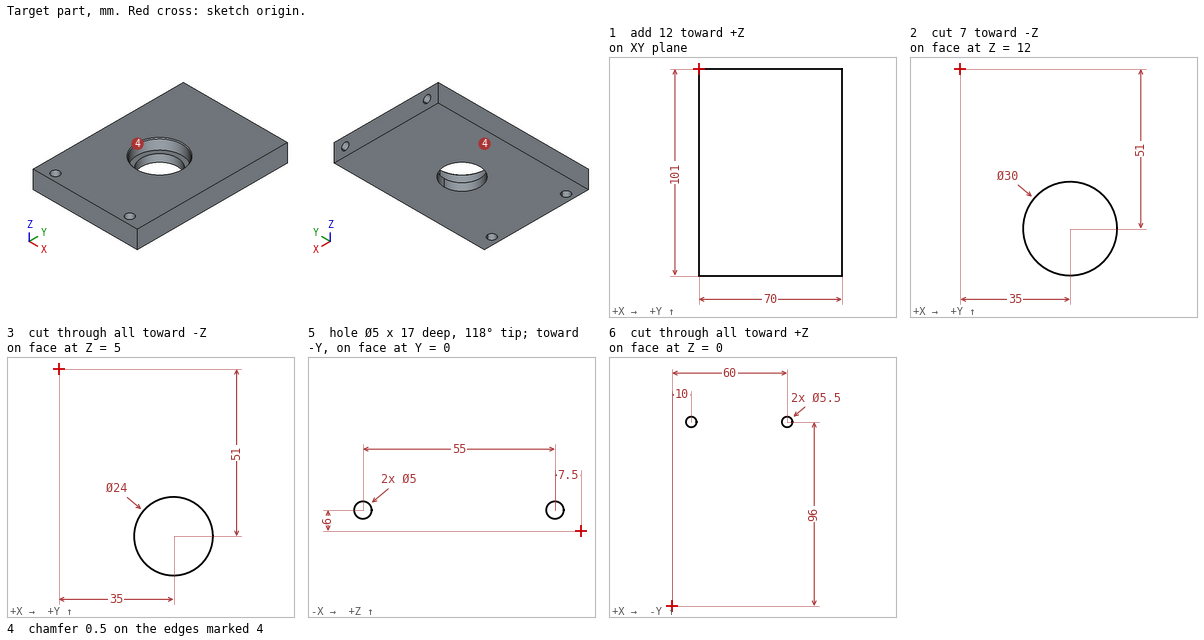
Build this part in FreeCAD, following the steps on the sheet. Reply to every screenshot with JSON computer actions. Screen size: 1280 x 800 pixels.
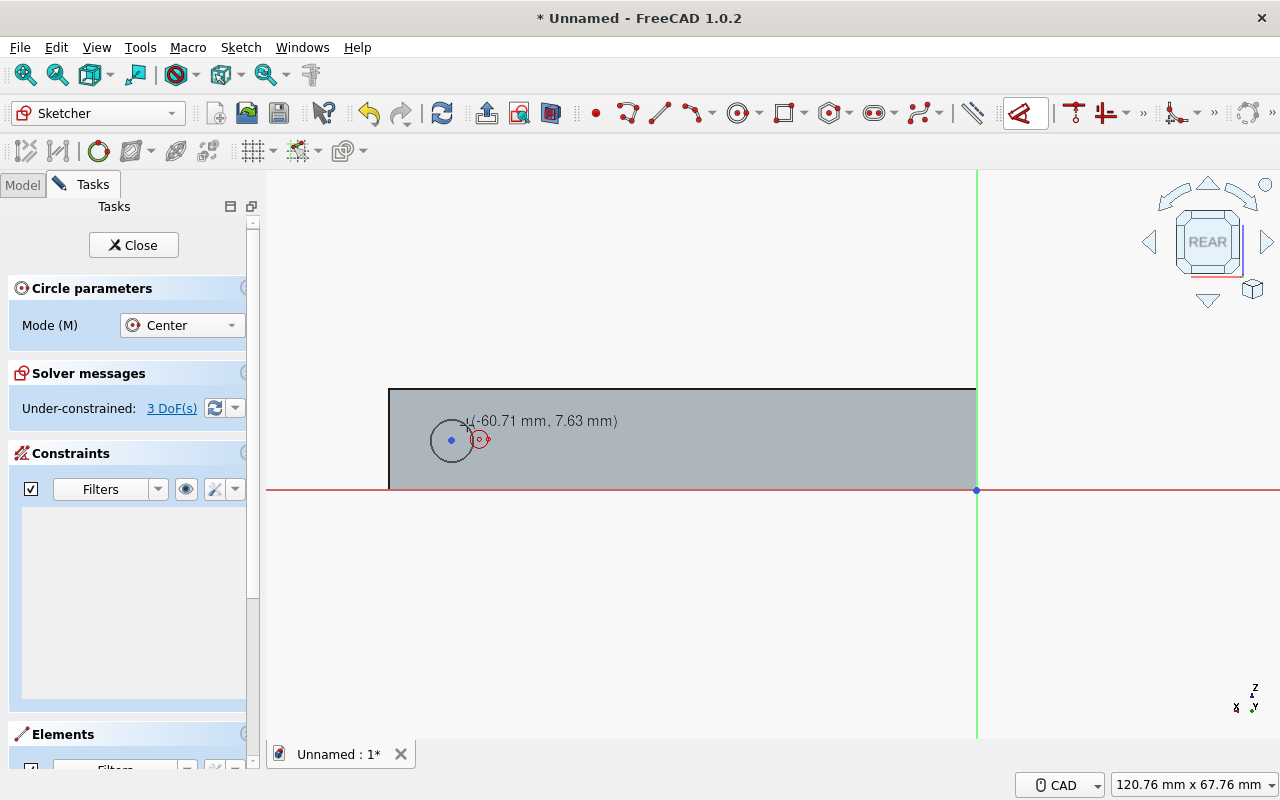
{"action": "left_click", "coordinate": [914, 440]}
{"action": "left_click", "coordinate": [929, 425]}
{"action": "key", "text": "Escape"}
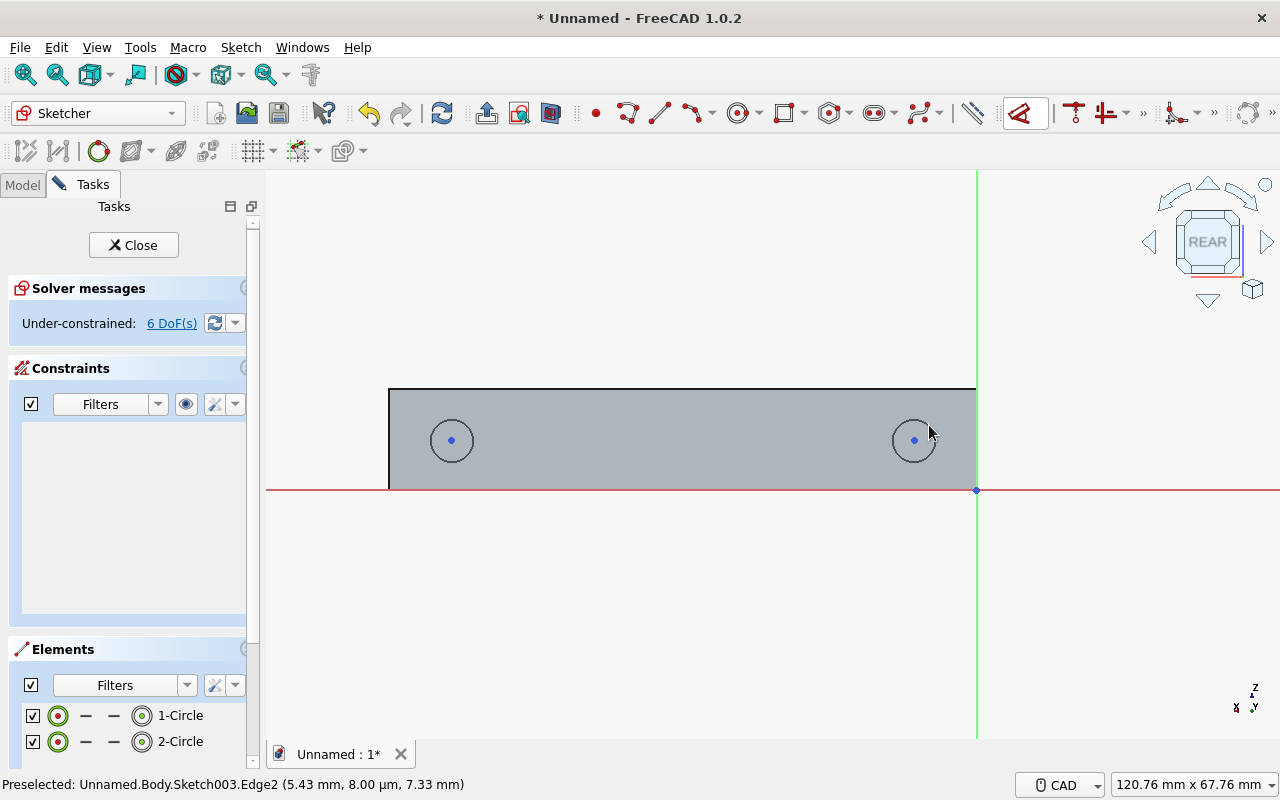
{"action": "left_click", "coordinate": [467, 426]}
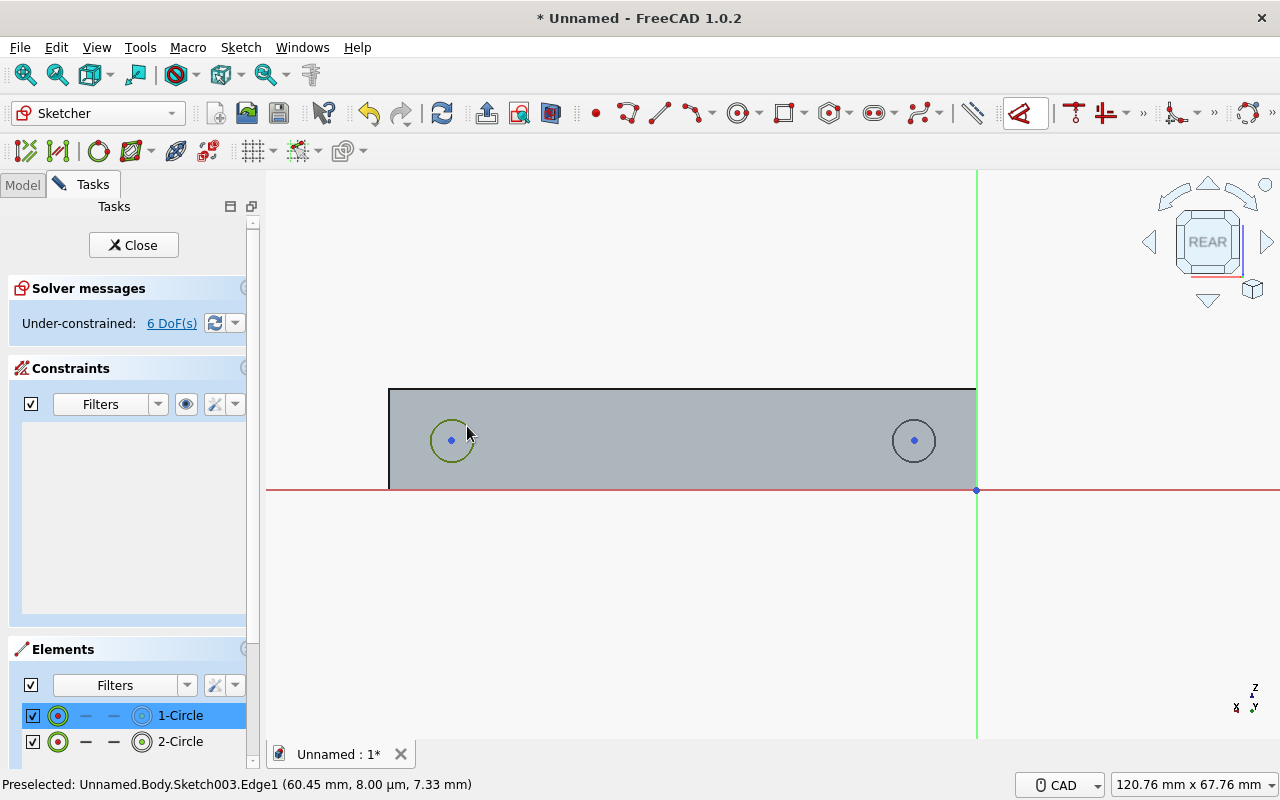
{"action": "left_click", "coordinate": [929, 426]}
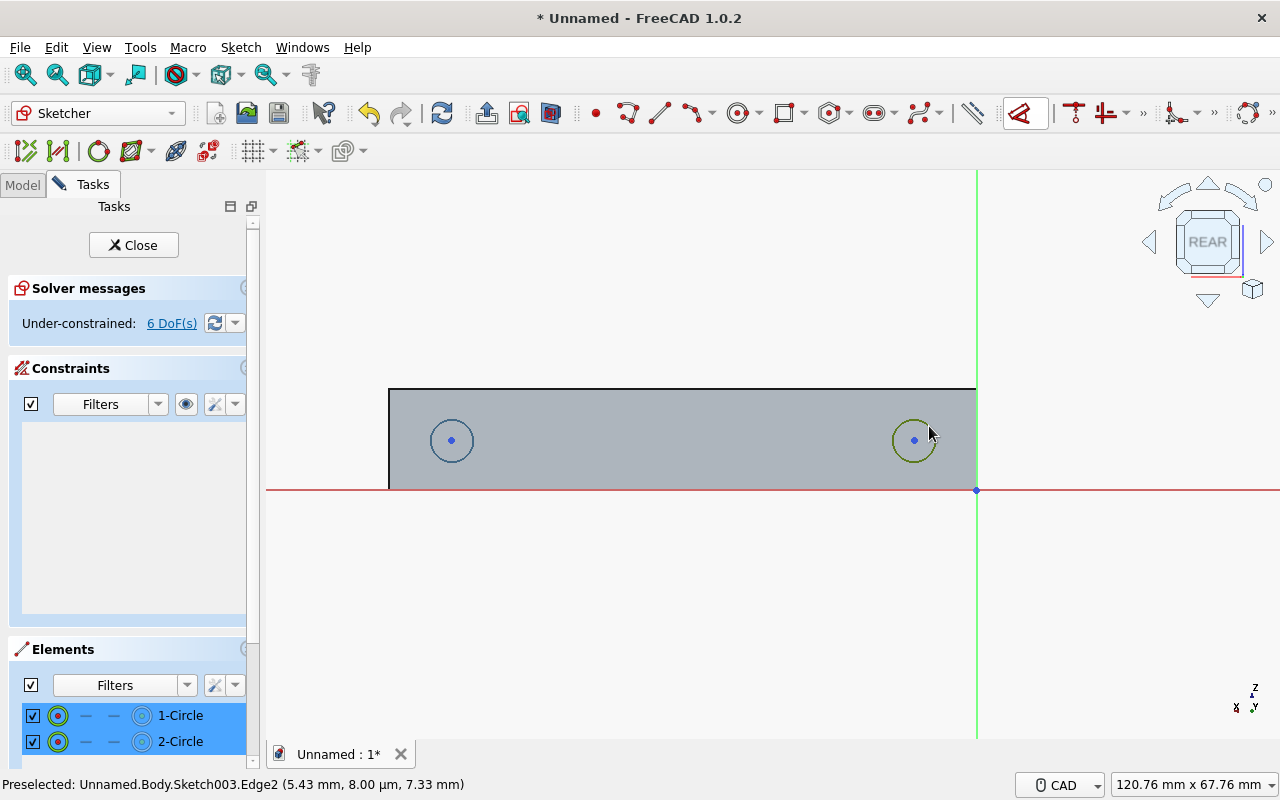
{"action": "key", "text": "e"}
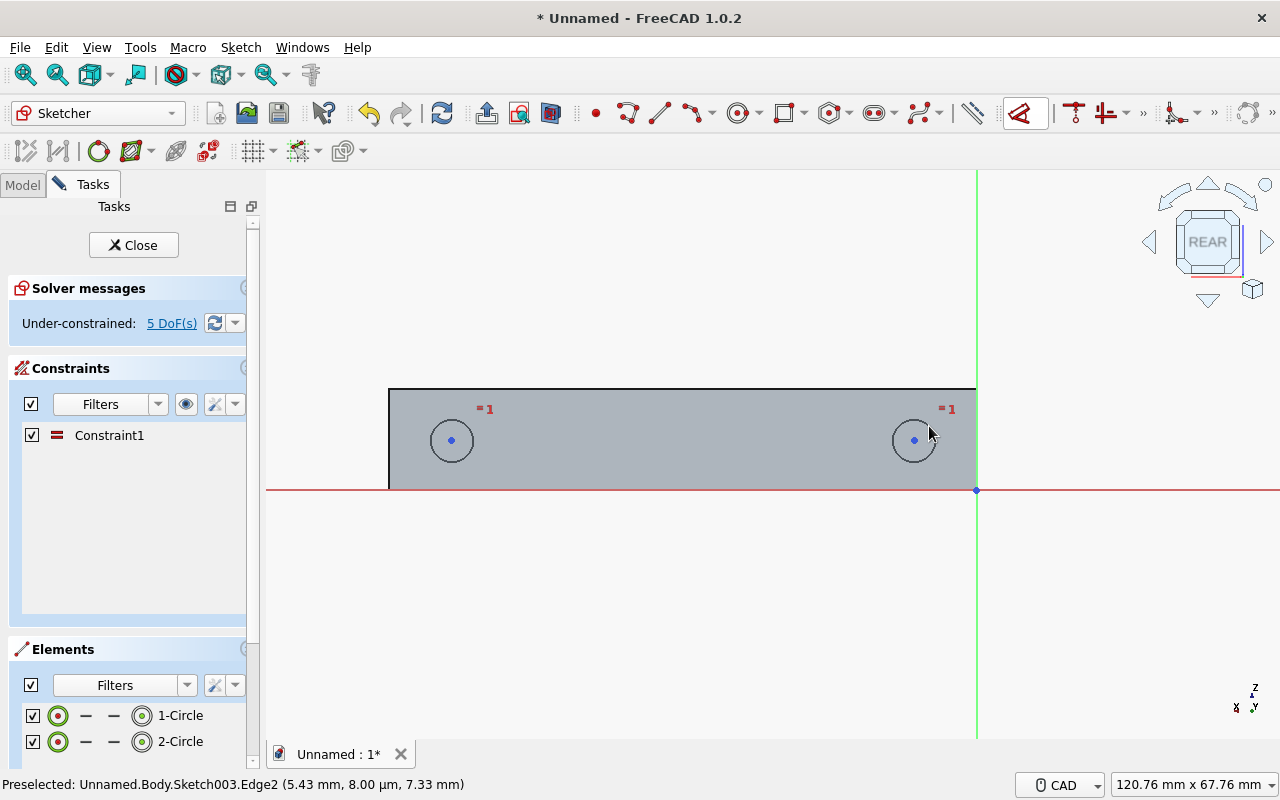
{"action": "left_click", "coordinate": [452, 441]}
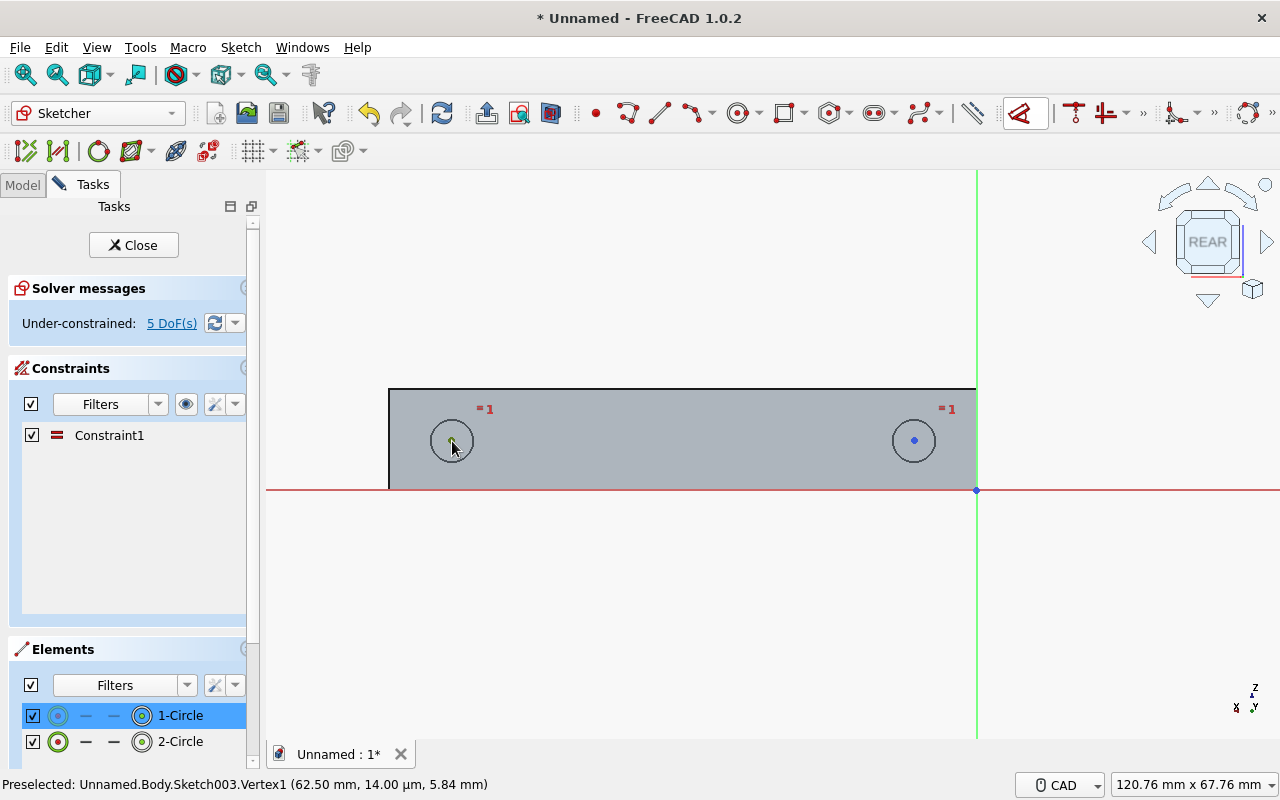
{"action": "left_click", "coordinate": [914, 441]}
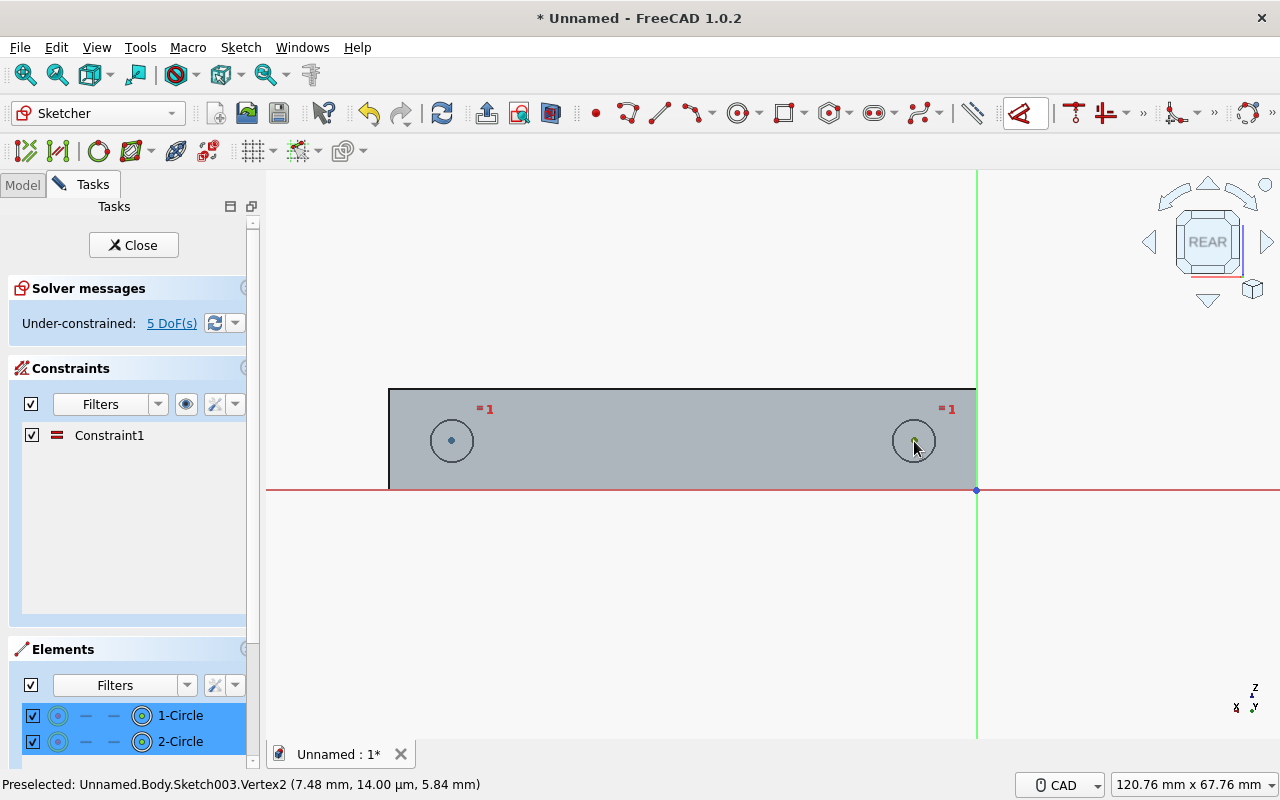
{"action": "left_click", "coordinate": [1128, 114]}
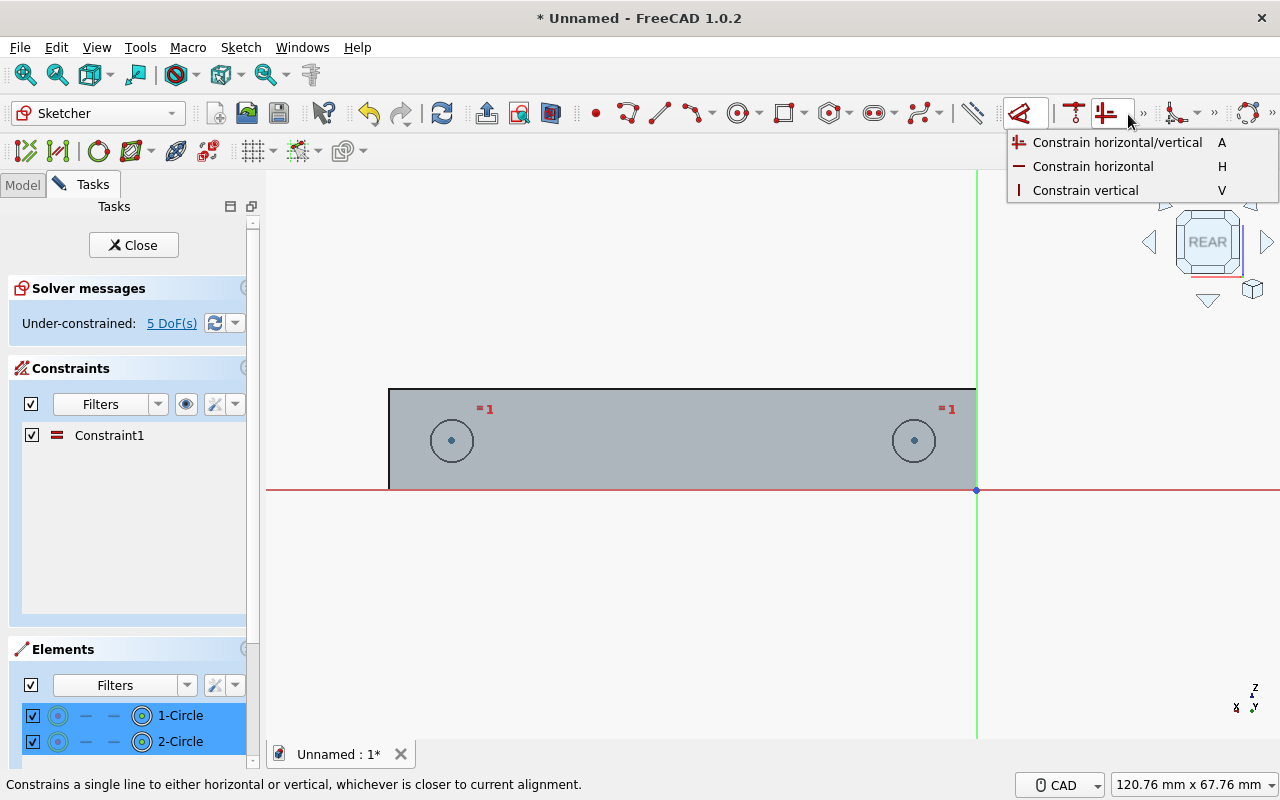
{"action": "left_click", "coordinate": [1143, 166]}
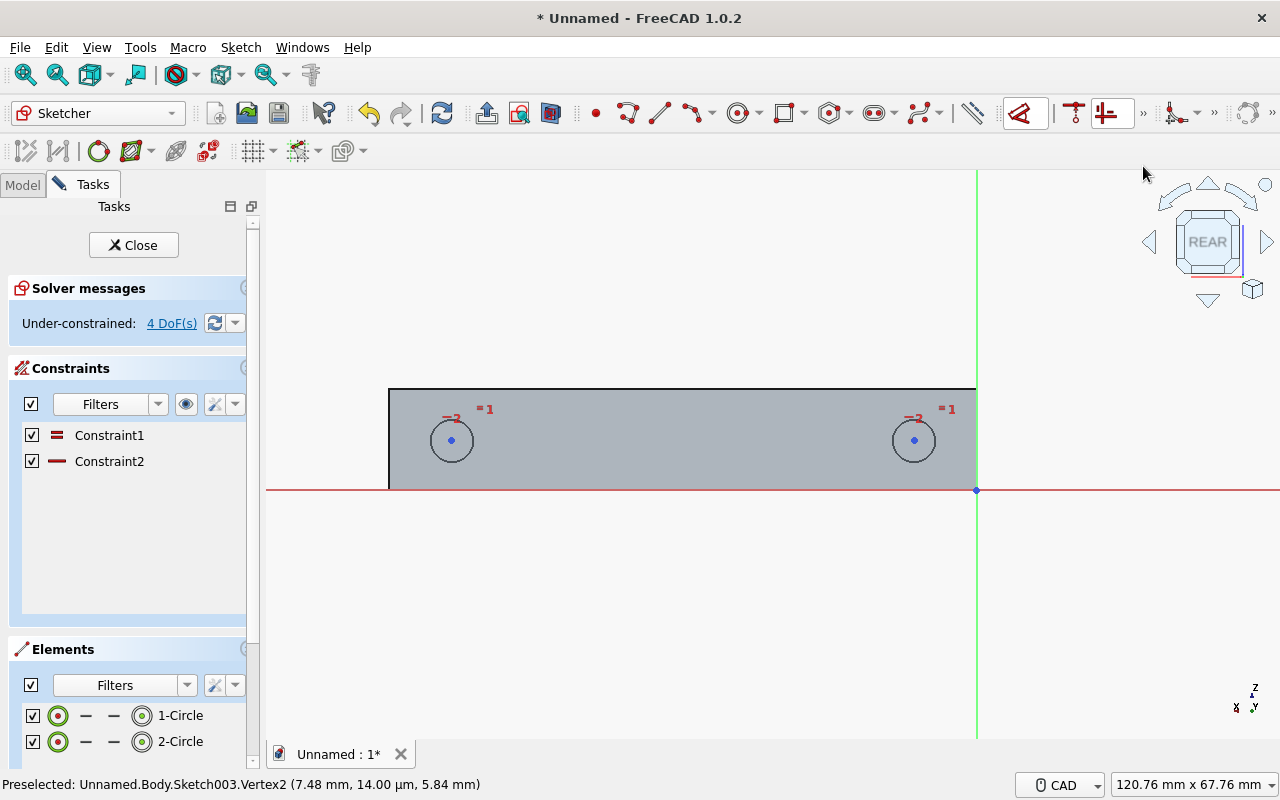
{"action": "left_click", "coordinate": [467, 426]}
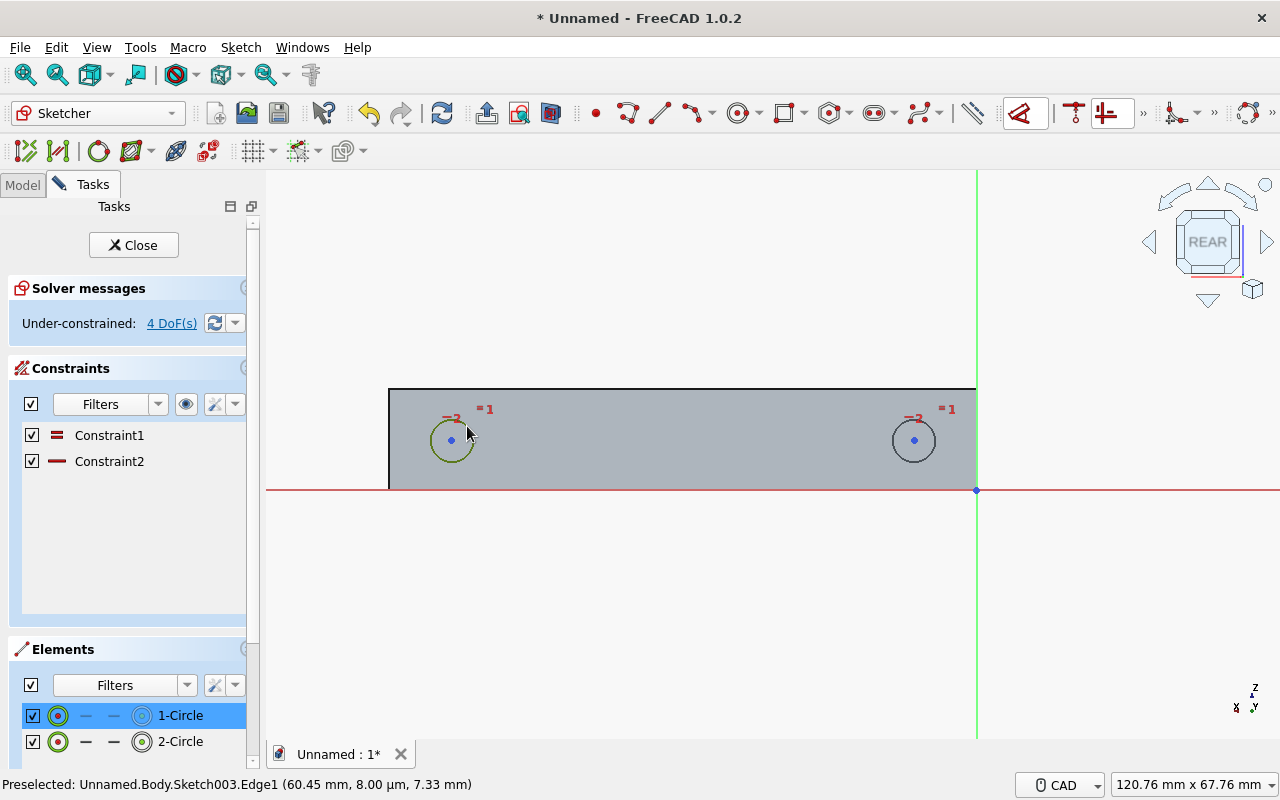
{"action": "key", "text": "k o"}